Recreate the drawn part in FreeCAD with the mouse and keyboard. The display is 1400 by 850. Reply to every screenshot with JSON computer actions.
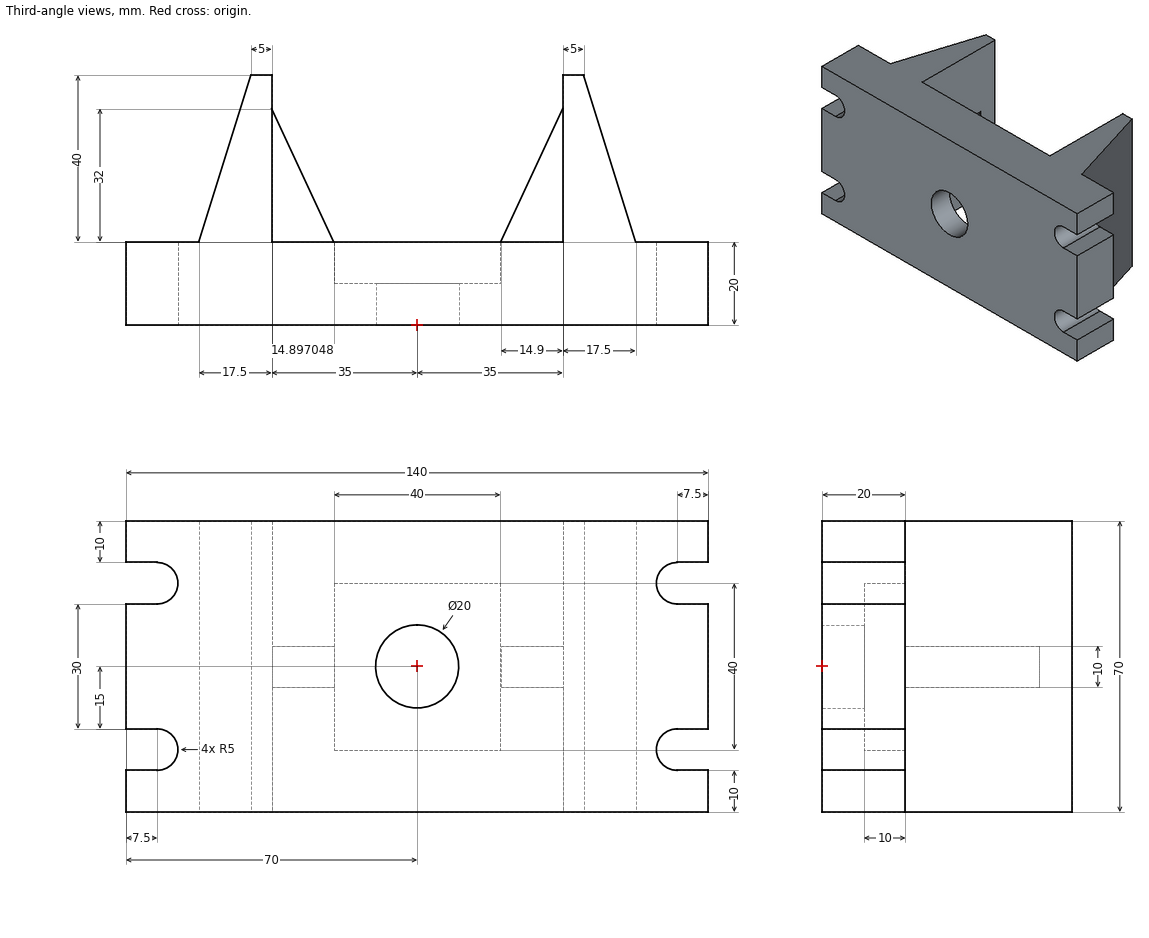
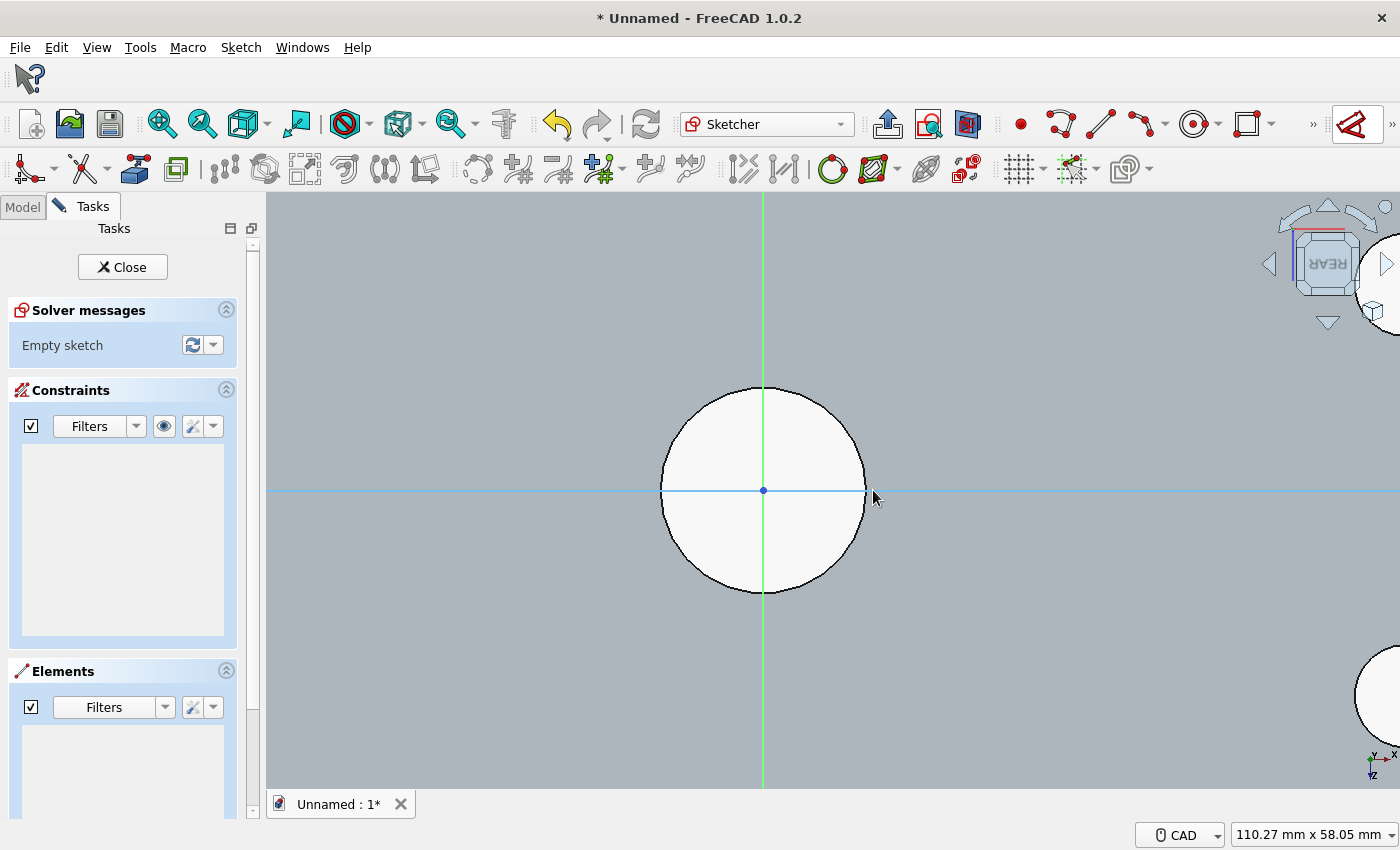
{"action": "key", "text": "g v"}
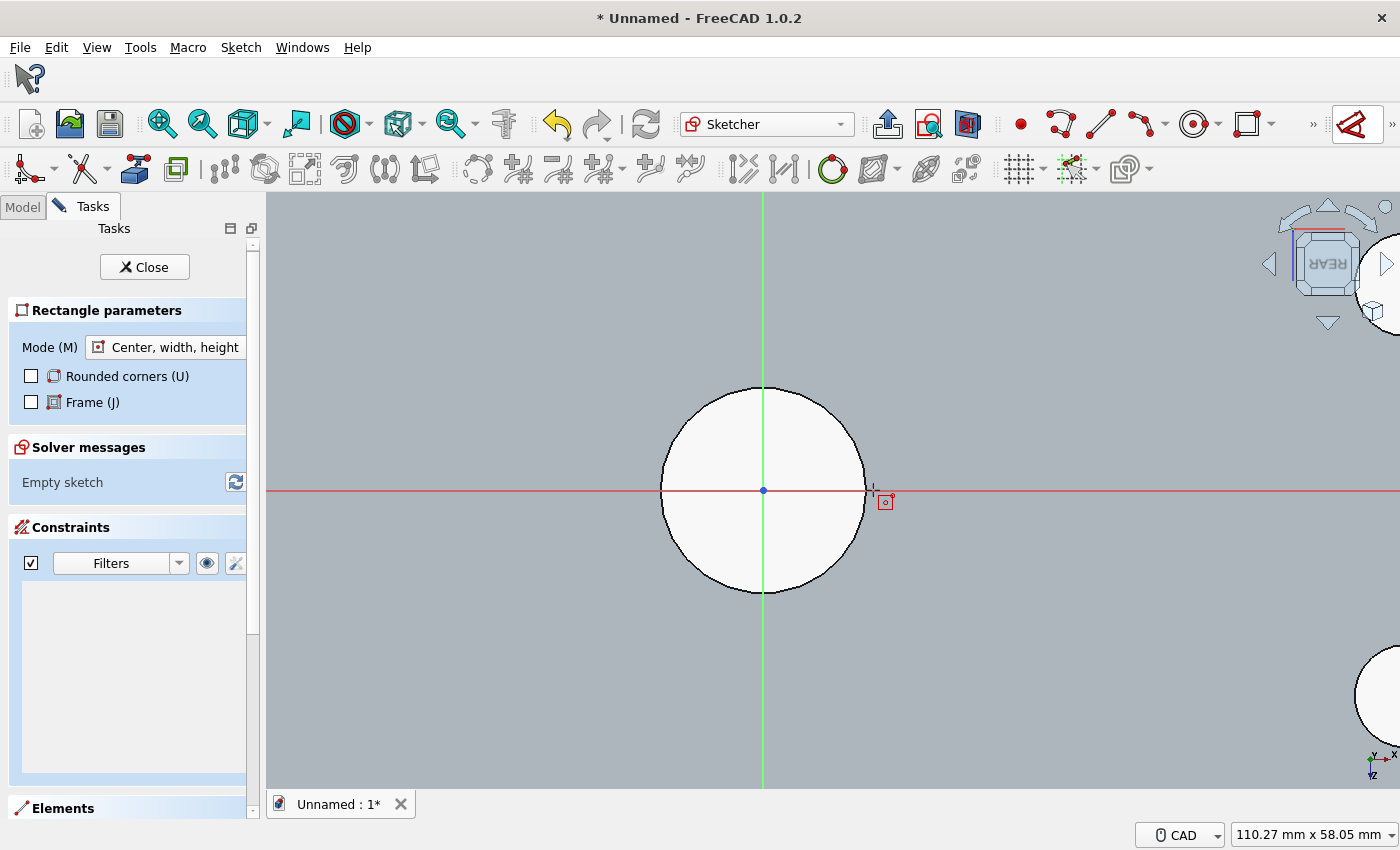
{"action": "left_click", "coordinate": [763, 490]}
{"action": "mouse_move", "coordinate": [969, 285]}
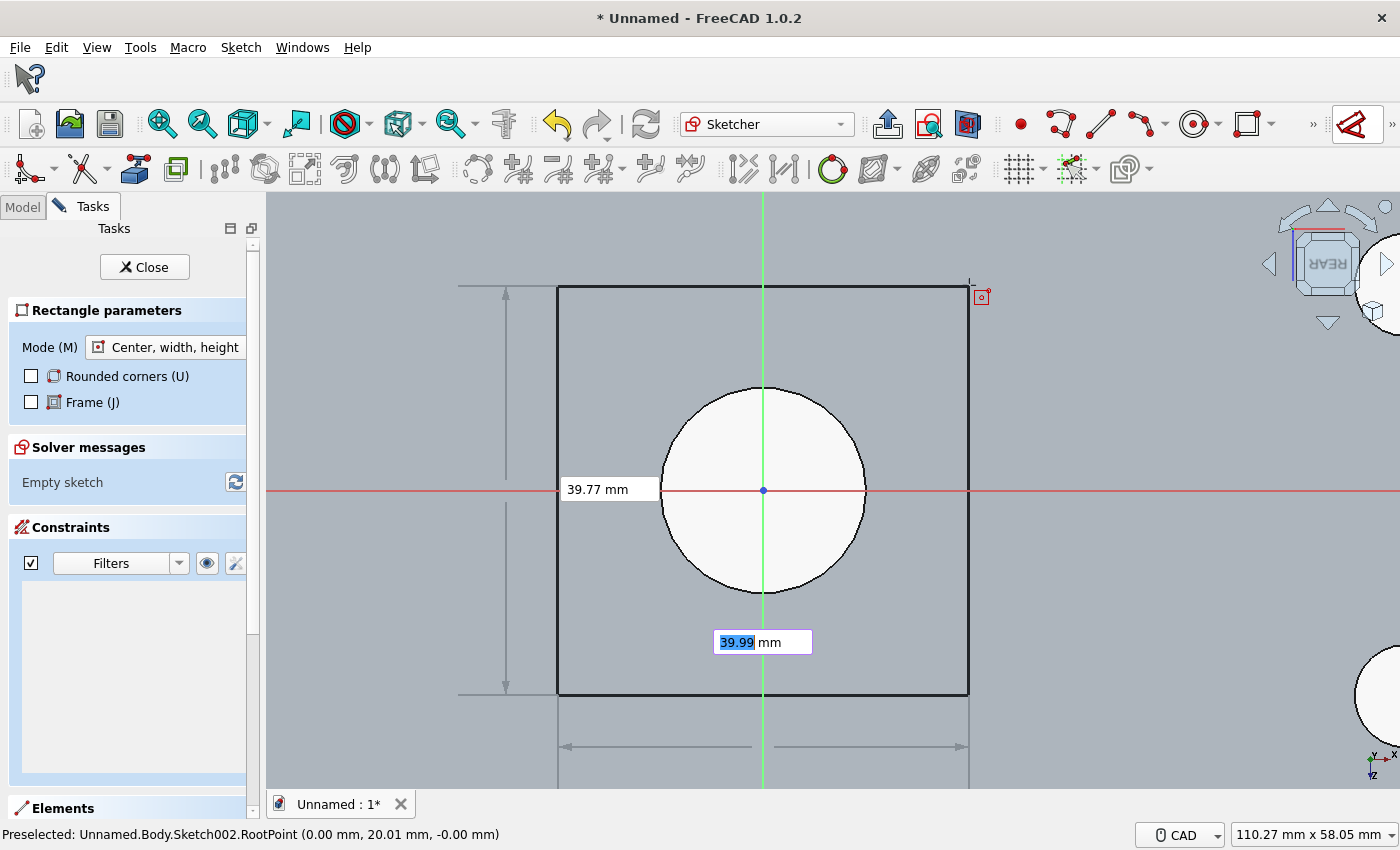
{"action": "type", "text": "40"}
{"action": "key", "text": "Tab"}
{"action": "type", "text": "40"}
{"action": "key", "text": "Return"}
{"action": "key", "text": "Escape"}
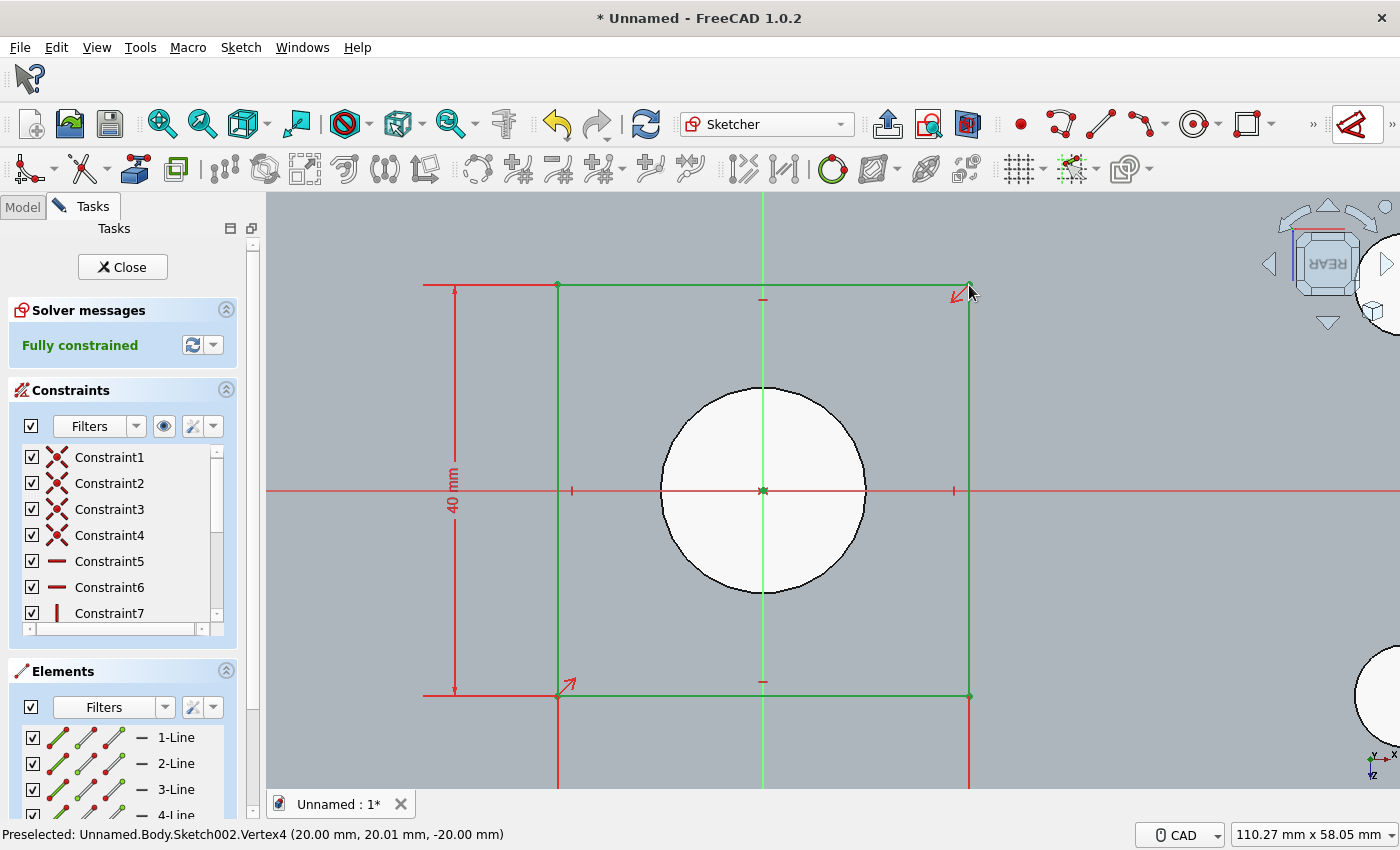
{"action": "left_click", "coordinate": [123, 267]}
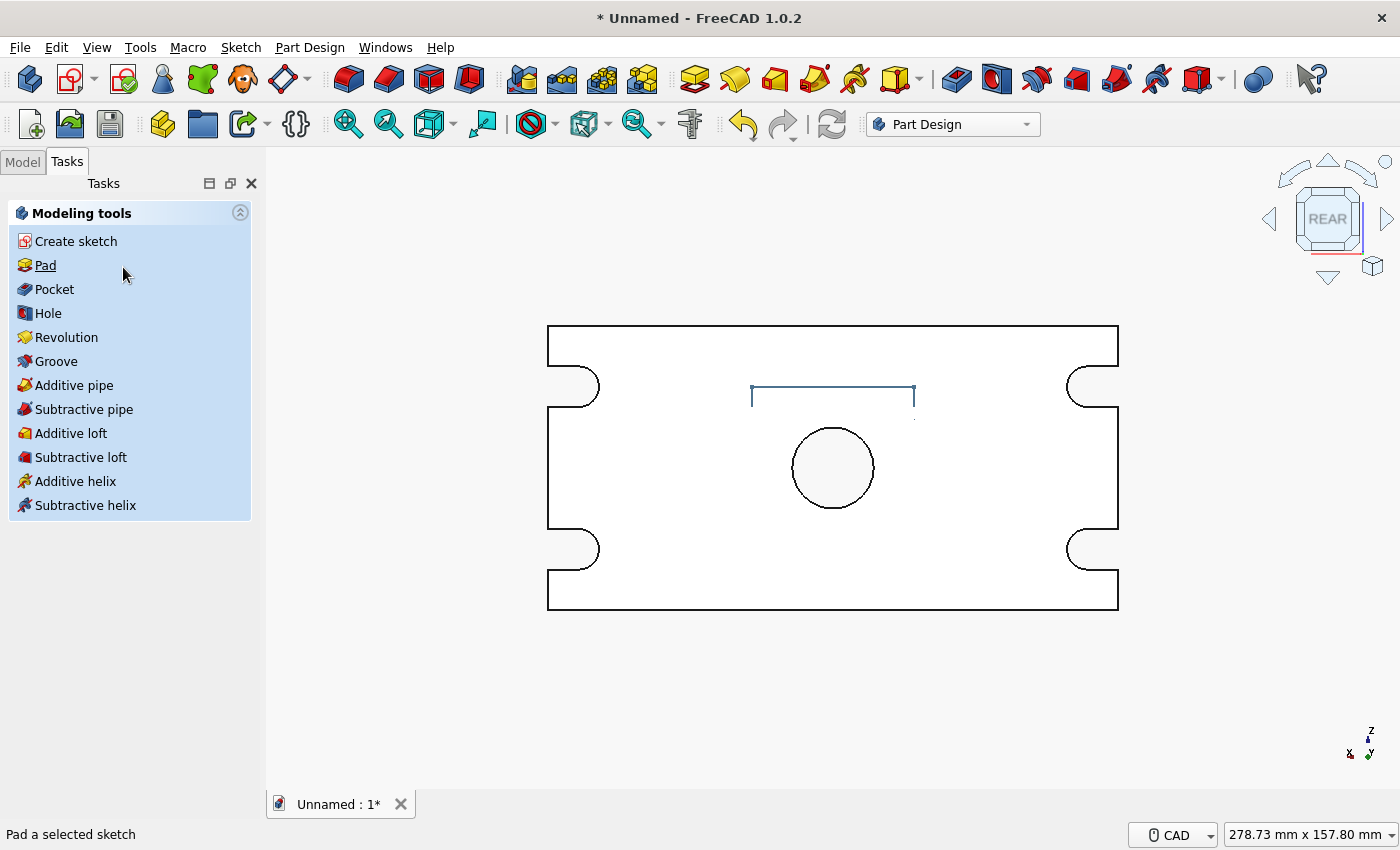
{"action": "left_click", "coordinate": [958, 80]}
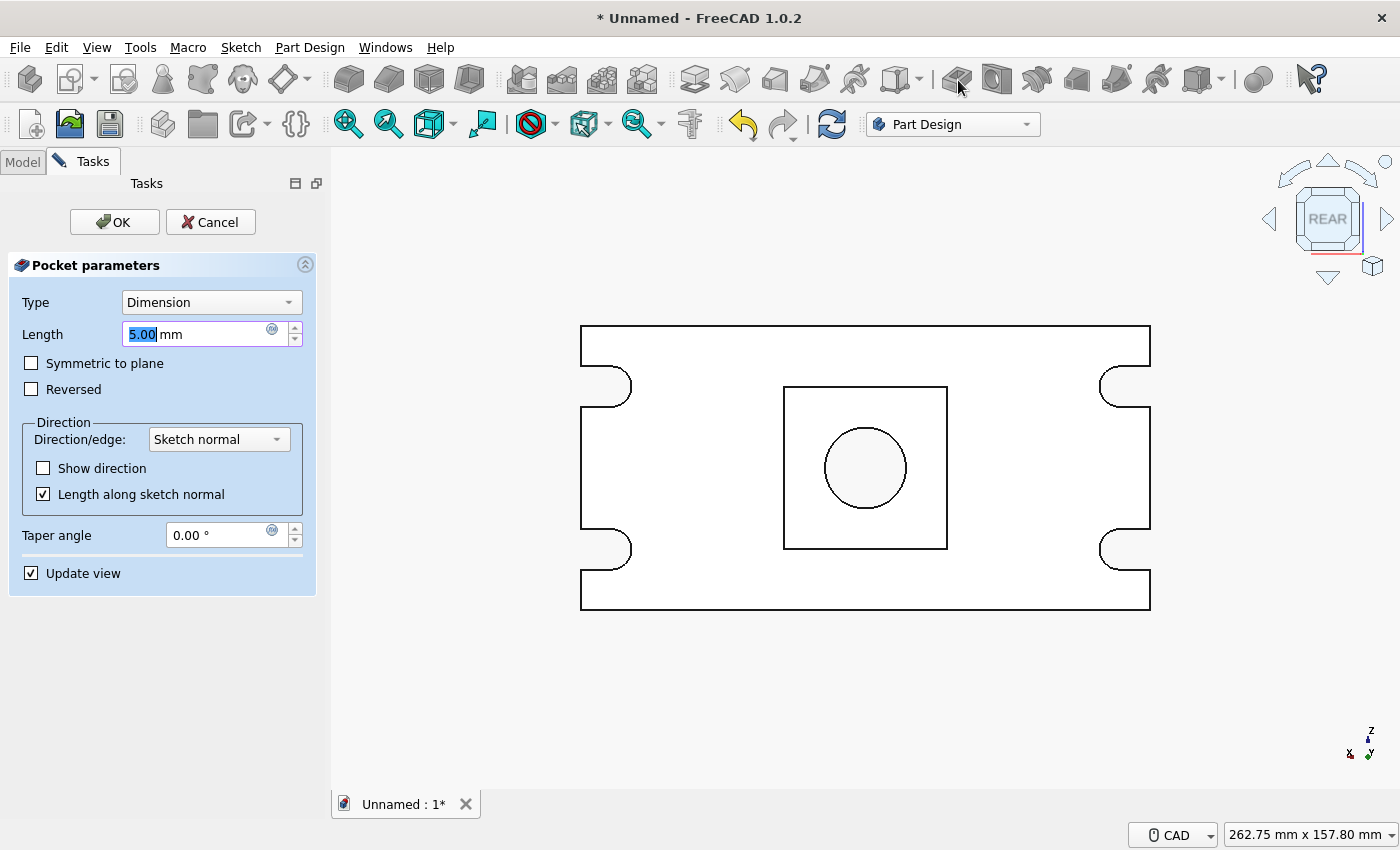
{"action": "type", "text": "10"}
{"action": "key", "text": "Tab"}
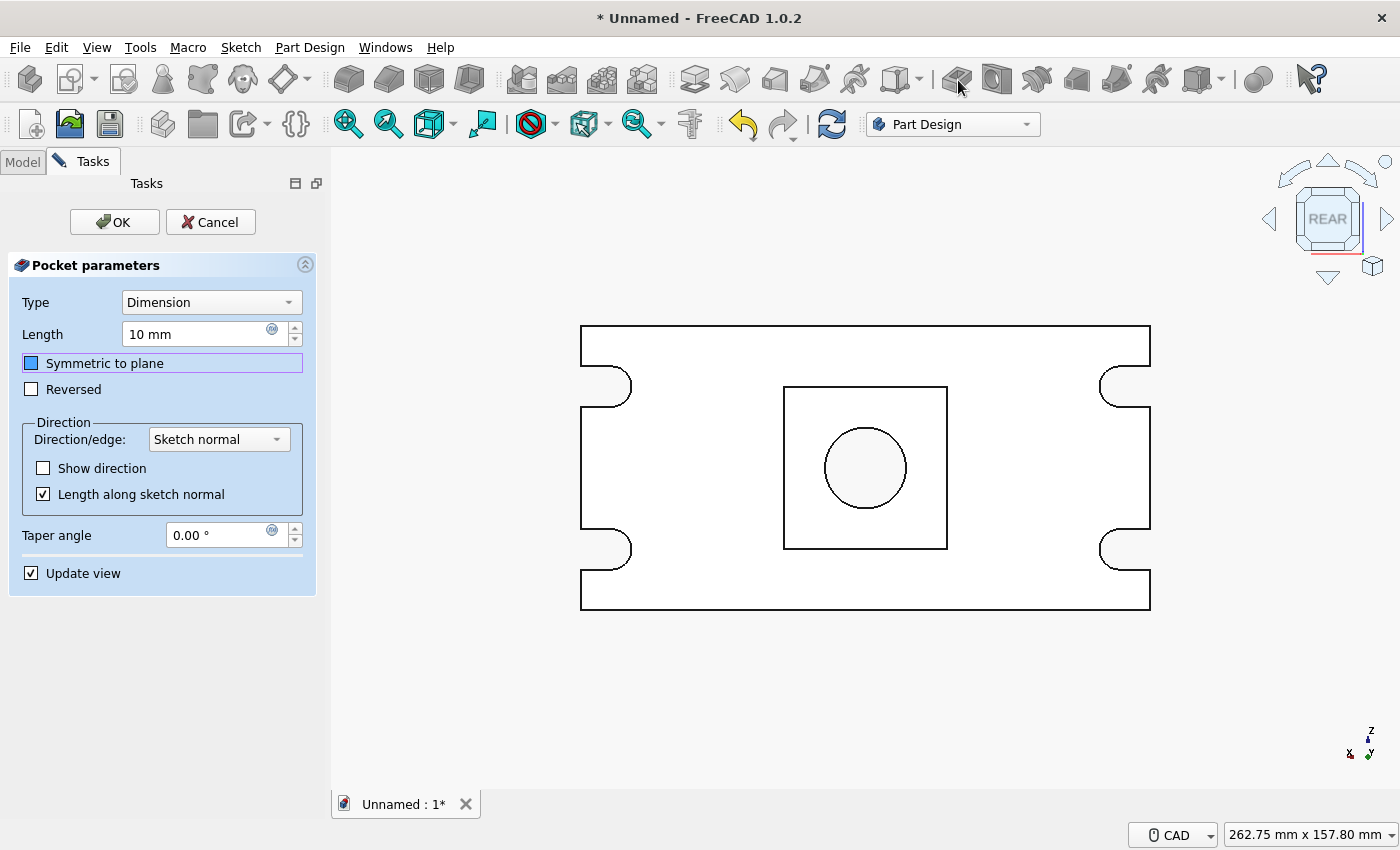
{"action": "left_click", "coordinate": [115, 222]}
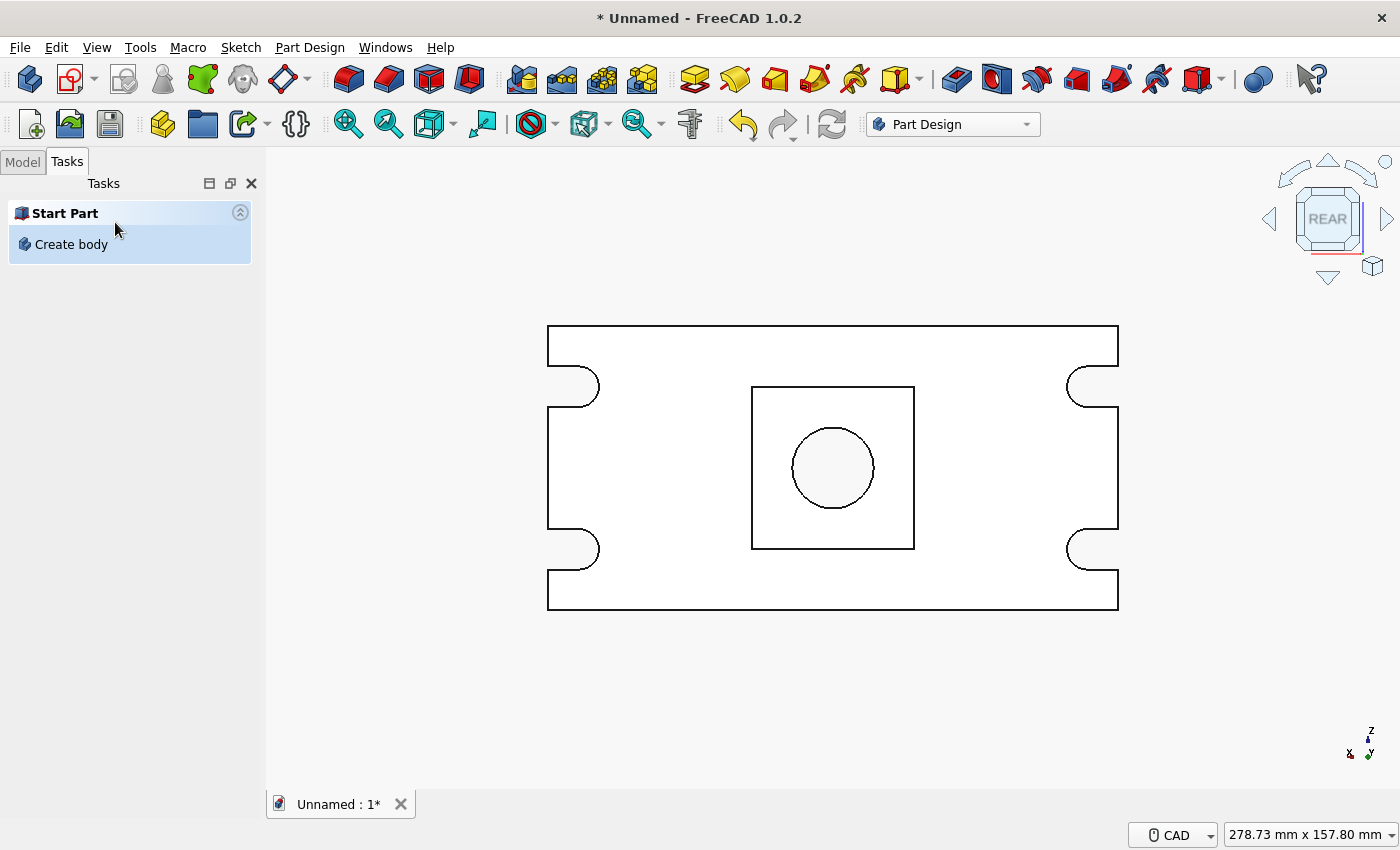
{"action": "key", "text": "0"}